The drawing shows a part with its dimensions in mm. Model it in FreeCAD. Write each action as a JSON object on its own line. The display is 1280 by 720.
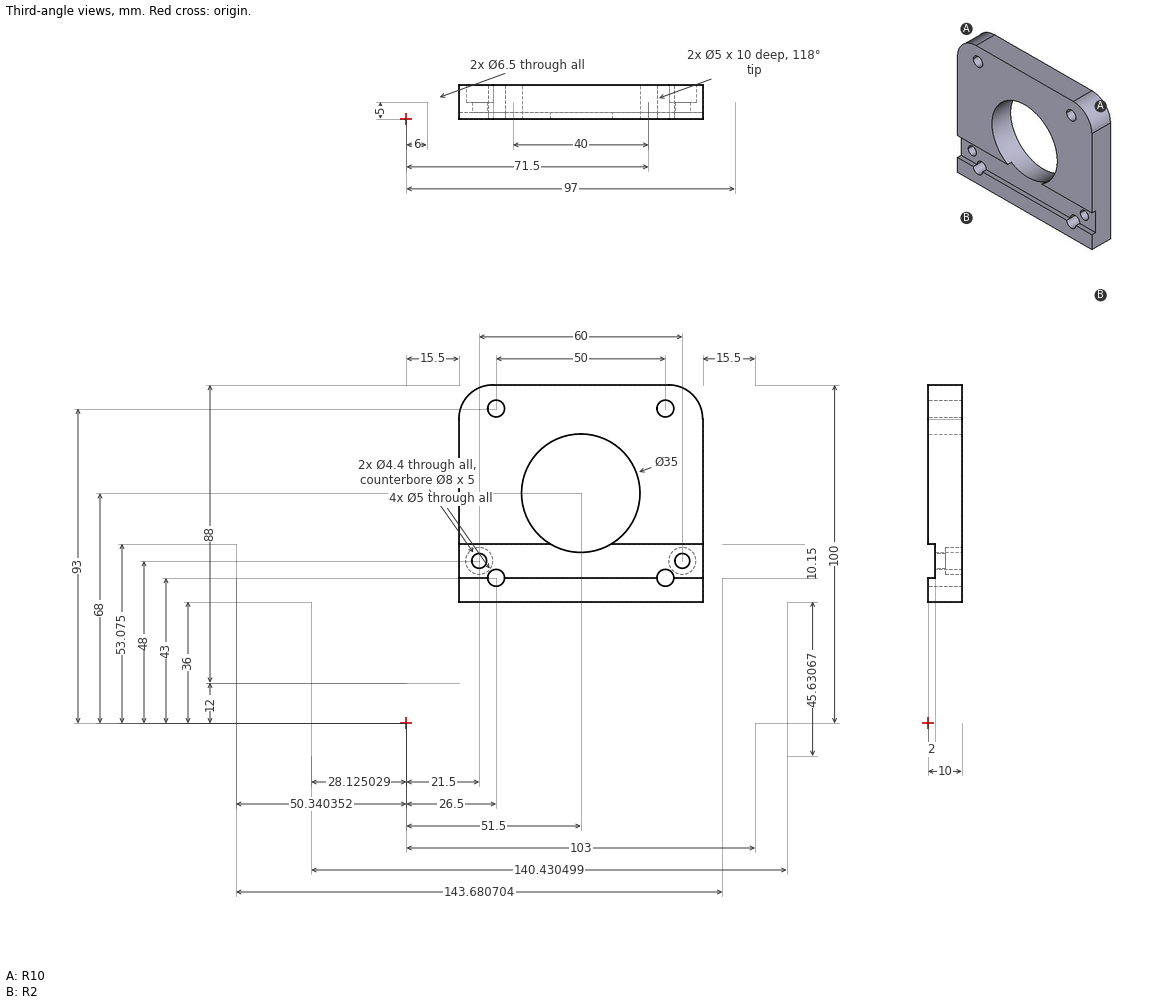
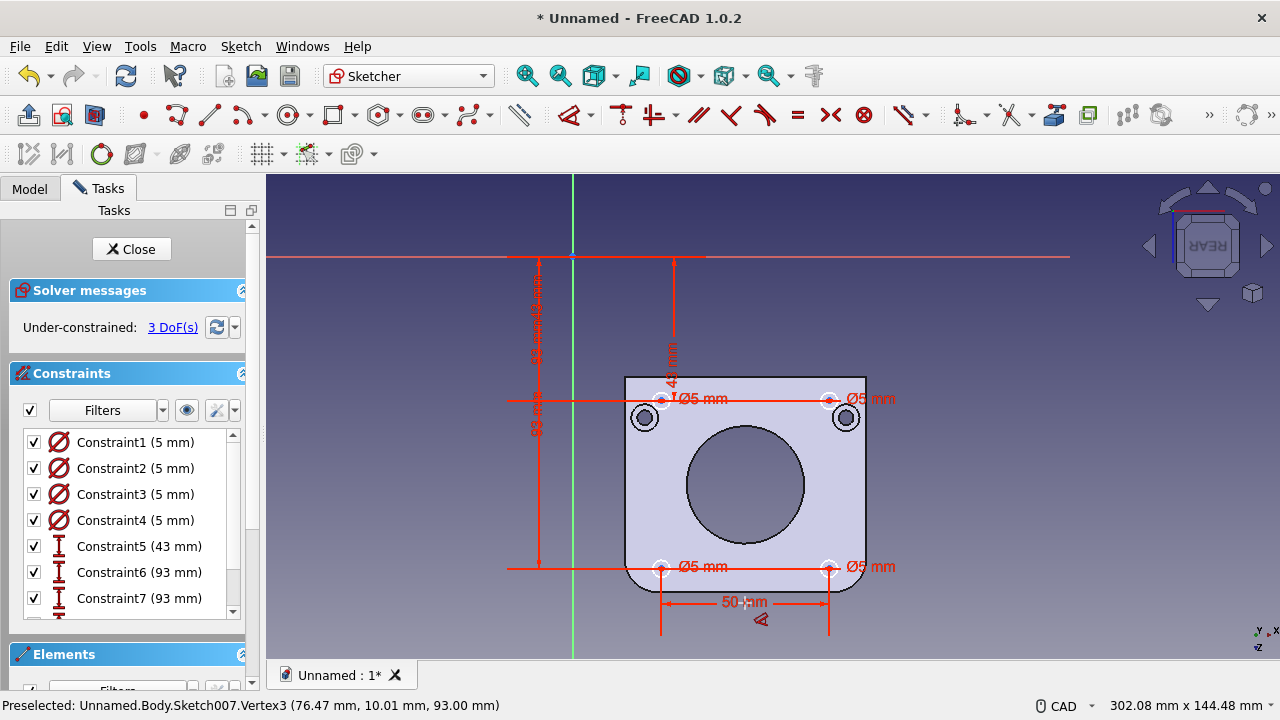
{"action": "left_click", "coordinate": [662, 401]}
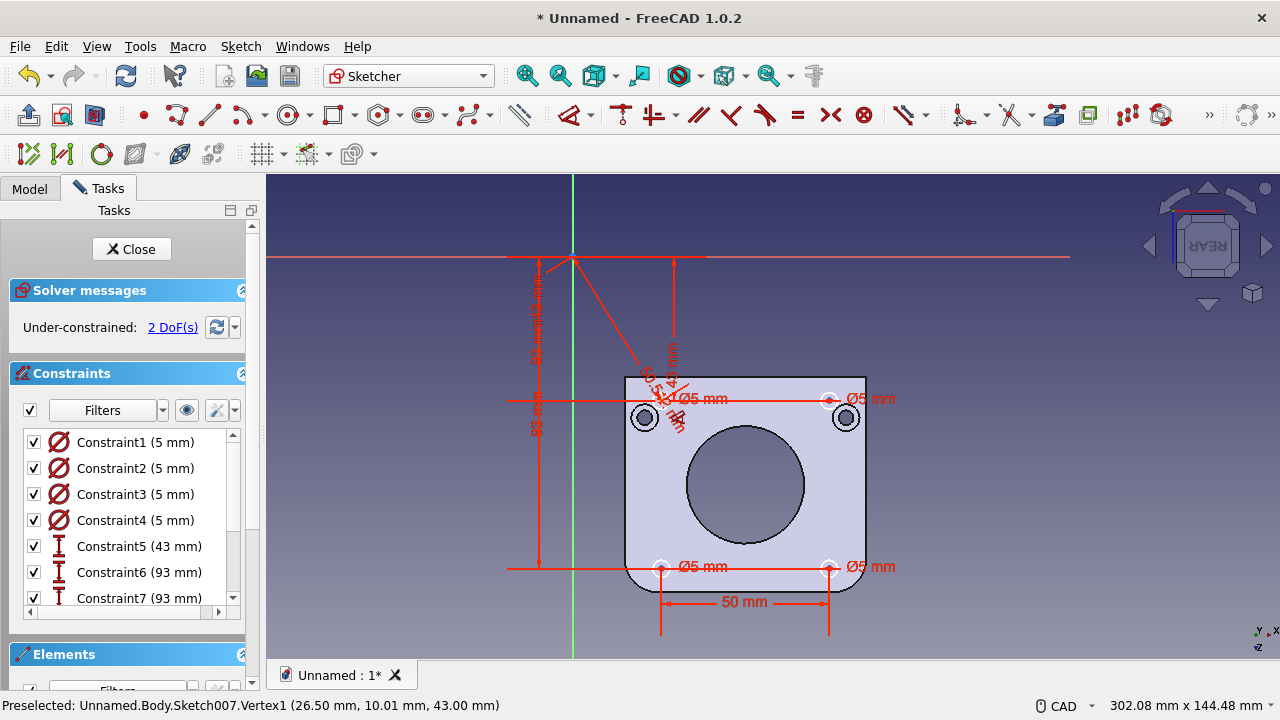
{"action": "left_click", "coordinate": [829, 569]}
{"action": "left_click", "coordinate": [745, 367]}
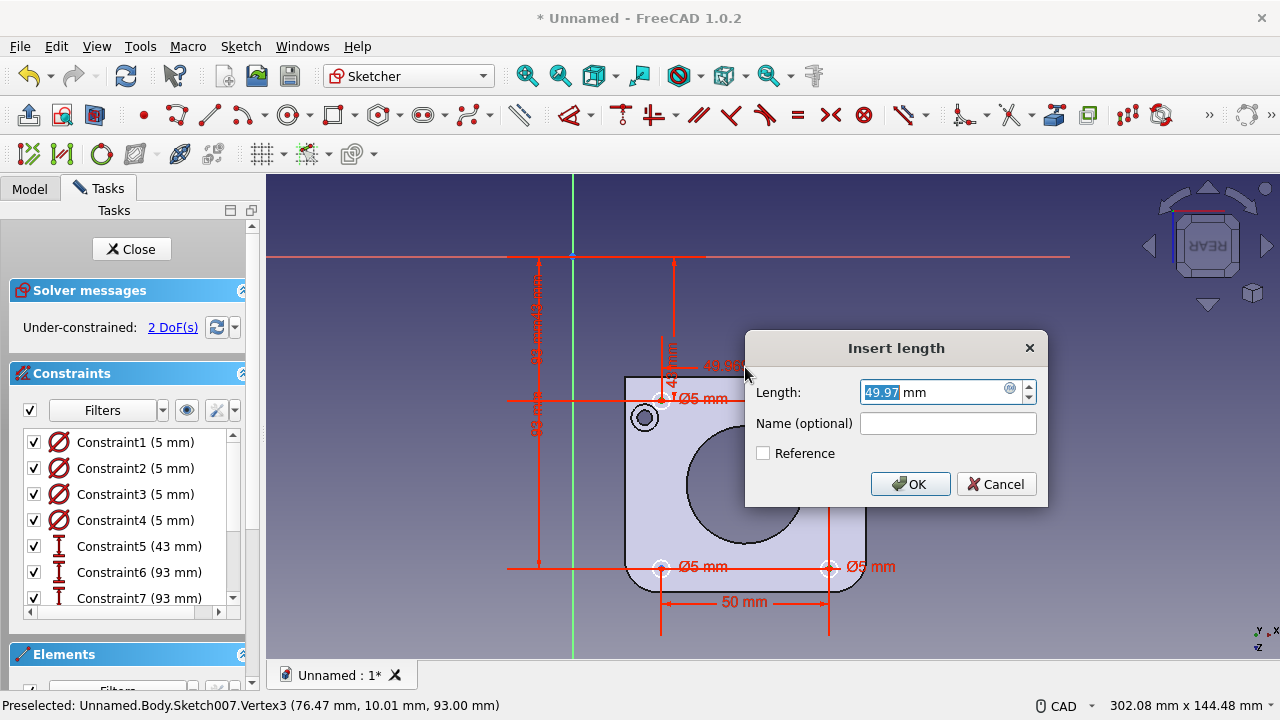
{"action": "type", "text": "50"}
{"action": "key", "text": "Return"}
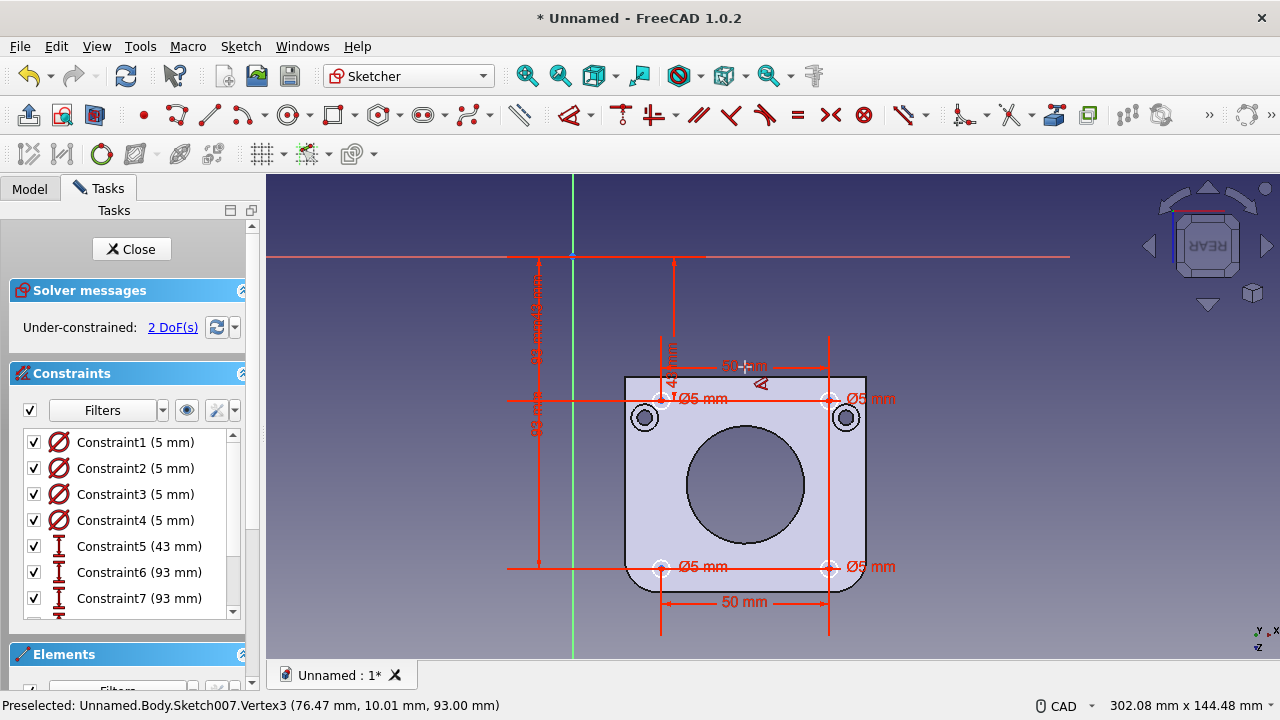
{"action": "left_click", "coordinate": [661, 401]}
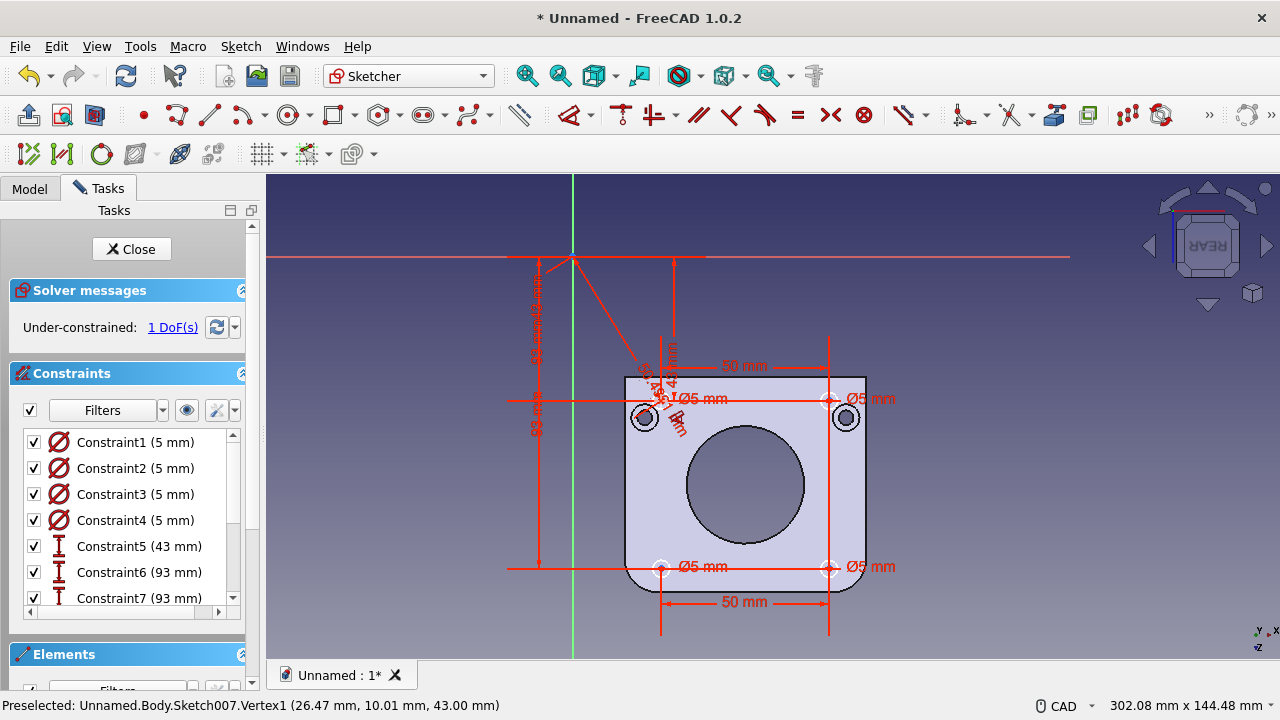
{"action": "left_click", "coordinate": [829, 401]}
{"action": "left_click", "coordinate": [745, 435]}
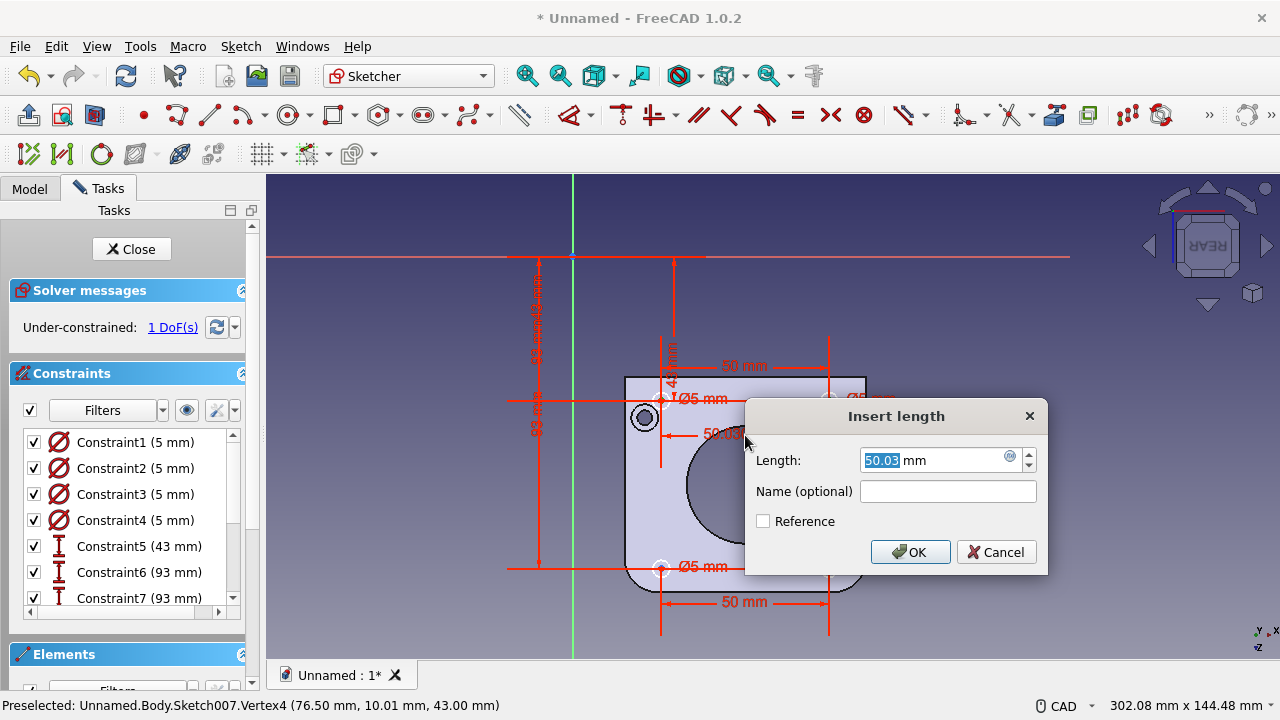
{"action": "type", "text": "50"}
{"action": "key", "text": "Return"}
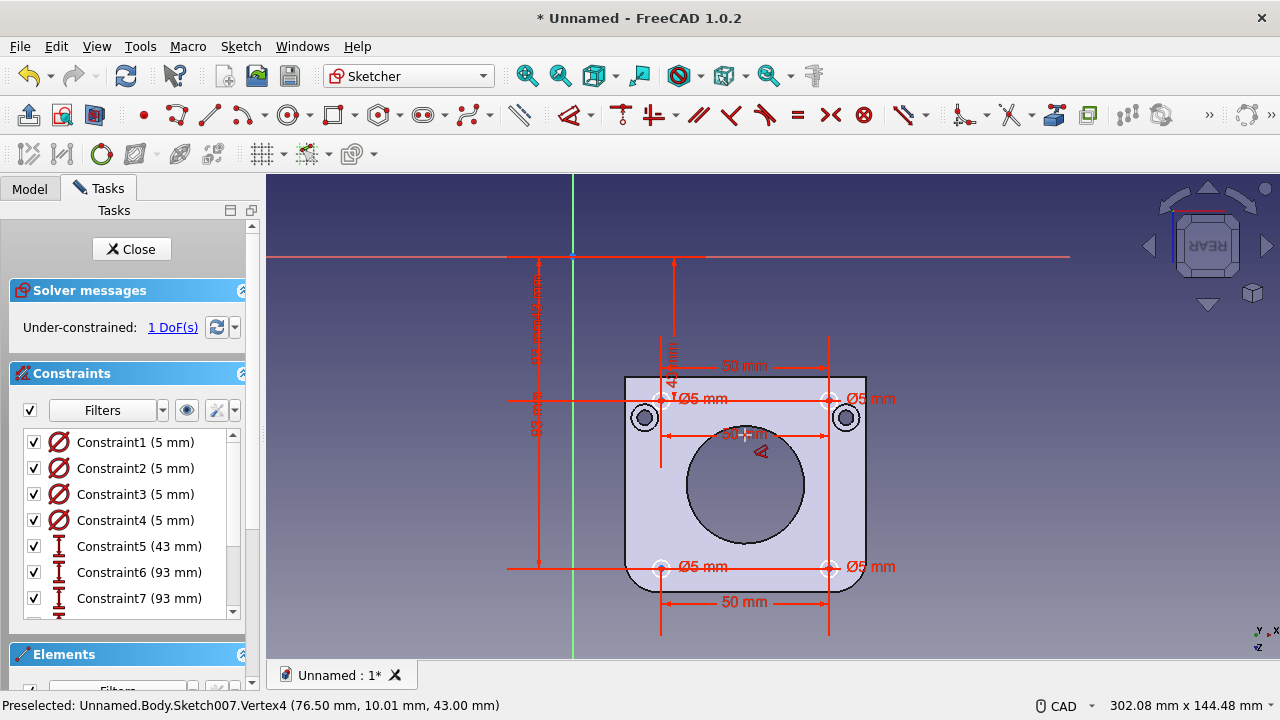
{"action": "left_click", "coordinate": [661, 401]}
{"action": "left_click", "coordinate": [617, 223]}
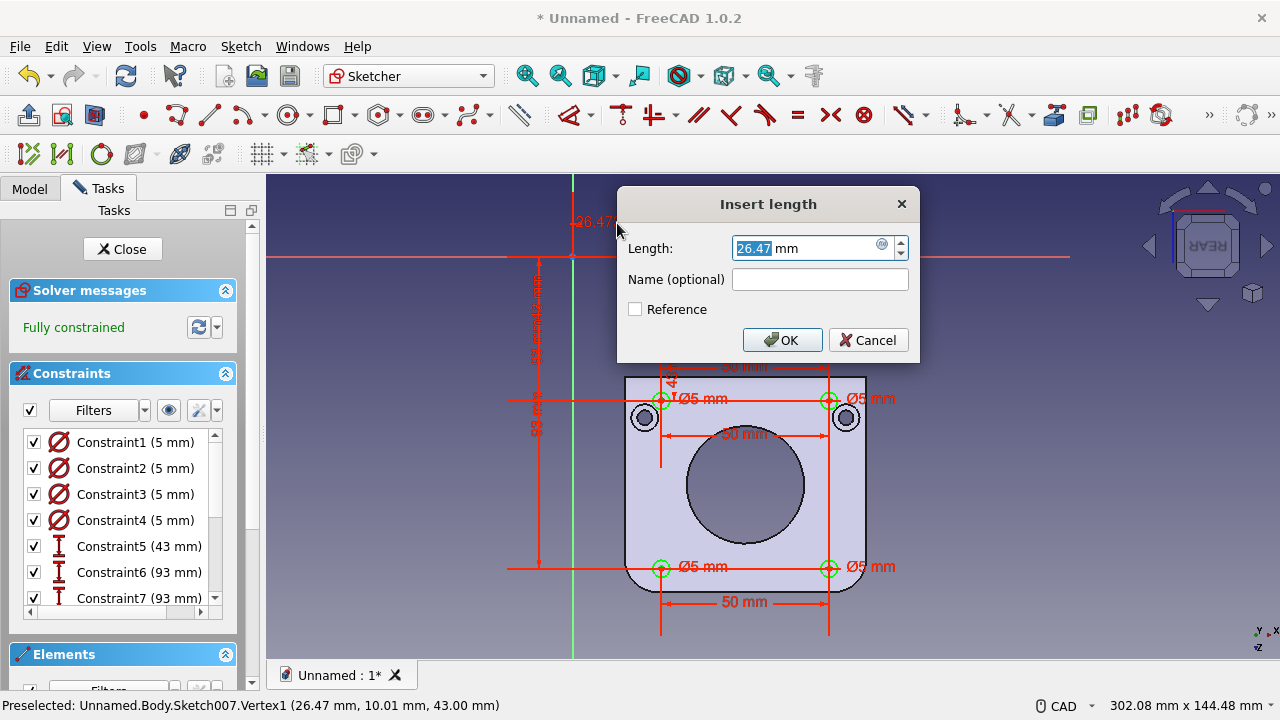
{"action": "type", "text": "26.5"}
{"action": "key", "text": "Return"}
{"action": "key", "text": "Escape"}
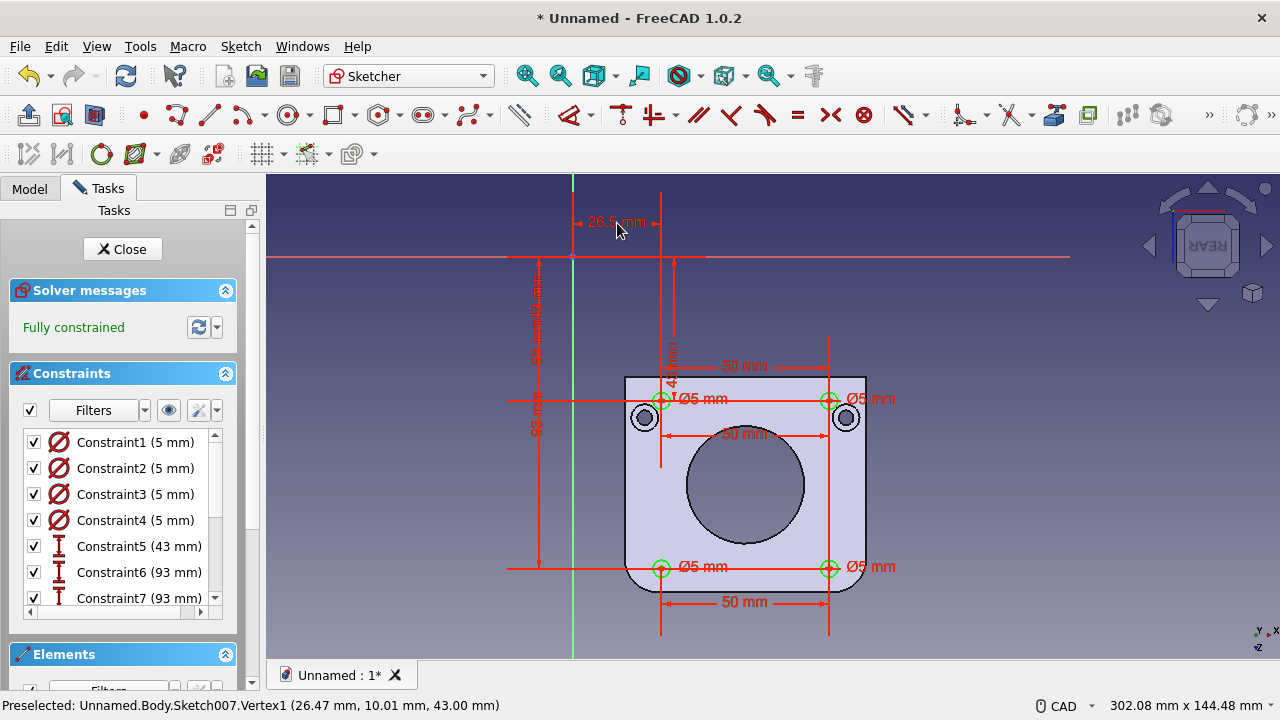
{"action": "left_click", "coordinate": [123, 249]}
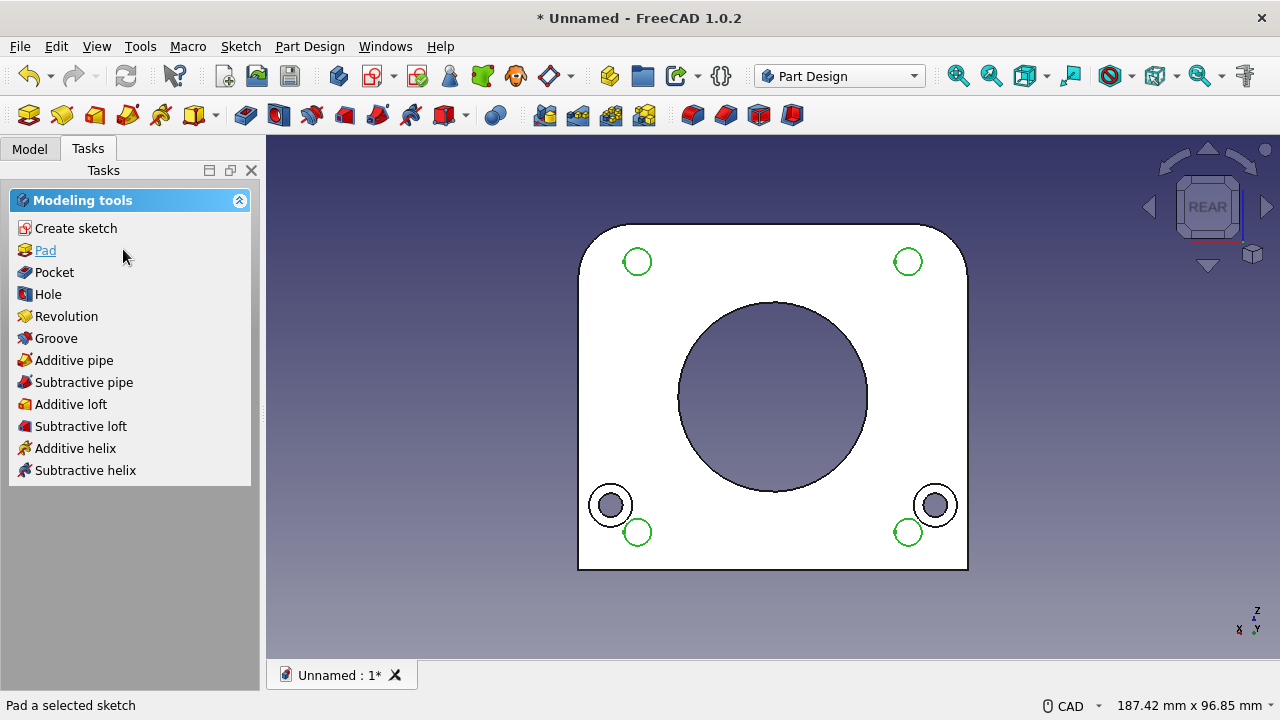
{"action": "left_click", "coordinate": [279, 116]}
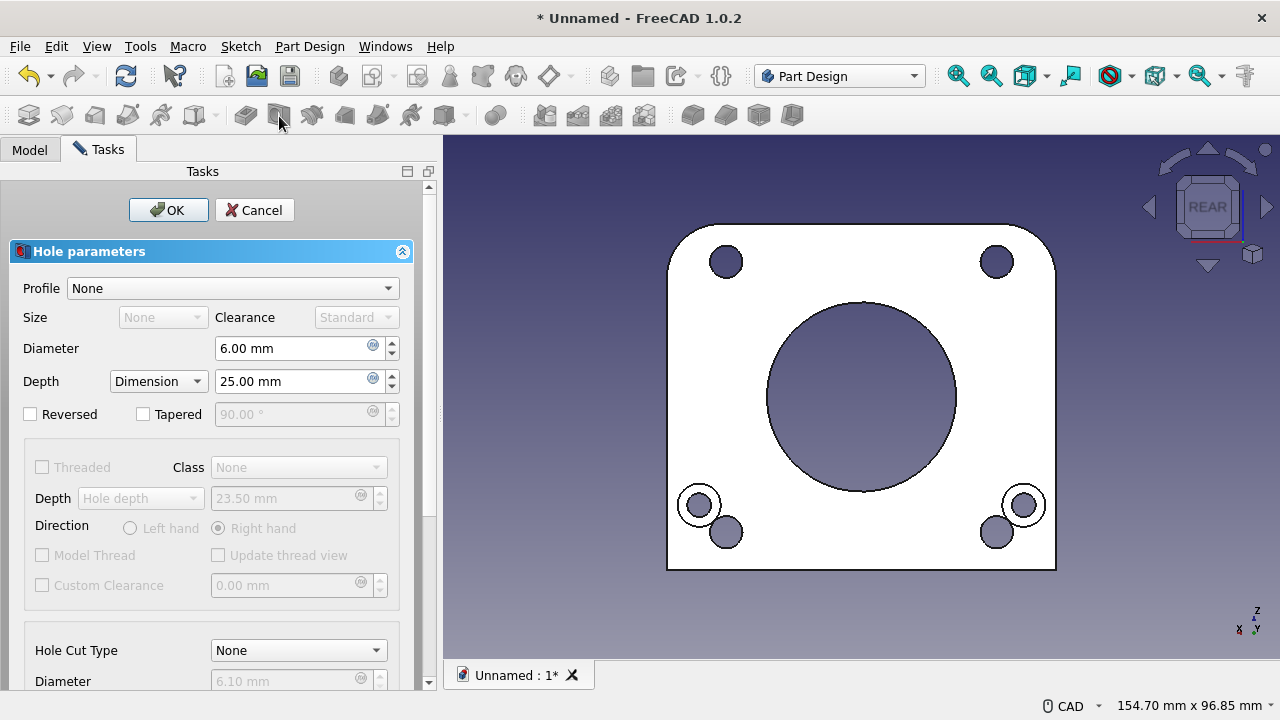
{"action": "triple_click", "coordinate": [300, 348]}